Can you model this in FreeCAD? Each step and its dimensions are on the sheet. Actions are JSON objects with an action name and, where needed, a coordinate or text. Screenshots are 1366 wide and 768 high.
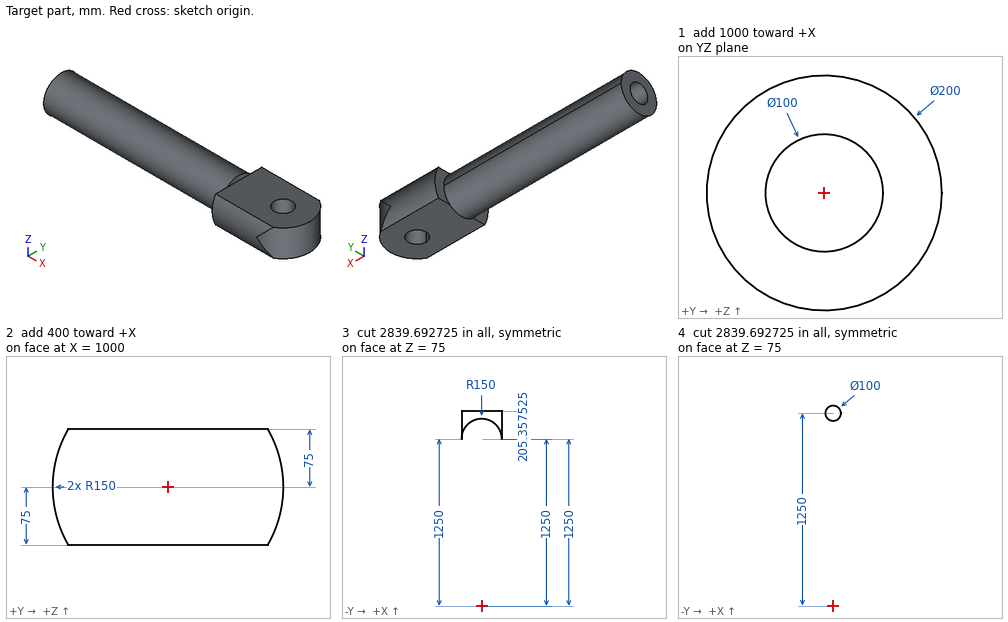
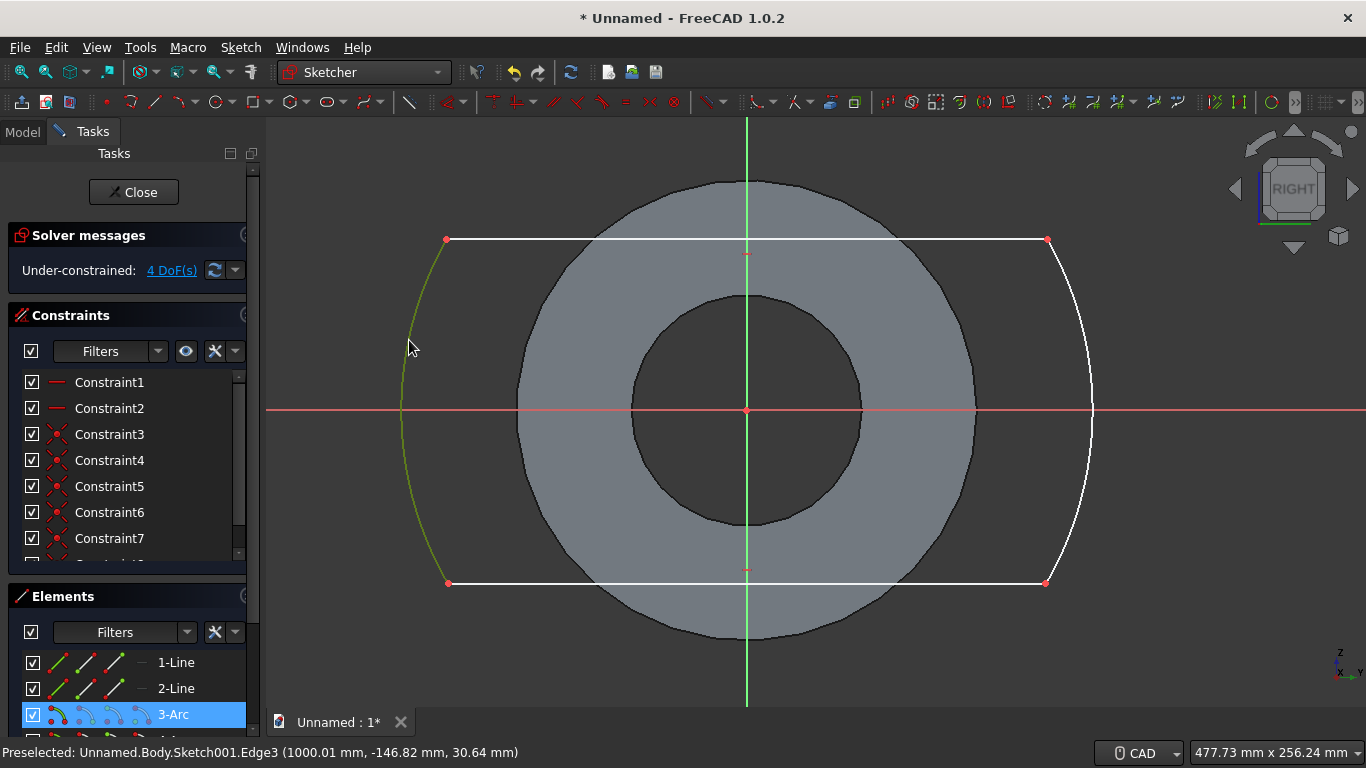
{"action": "left_click", "coordinate": [1085, 483]}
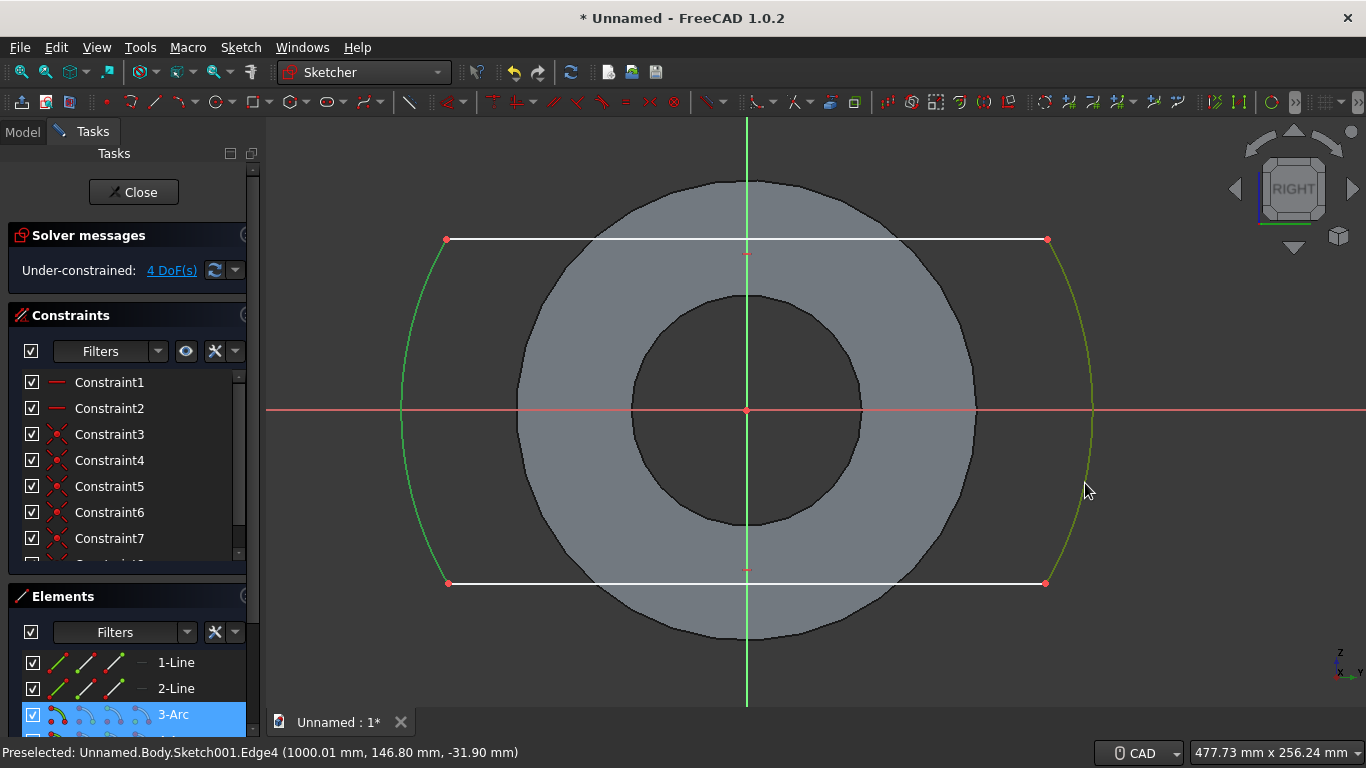
{"action": "left_click", "coordinate": [626, 102]}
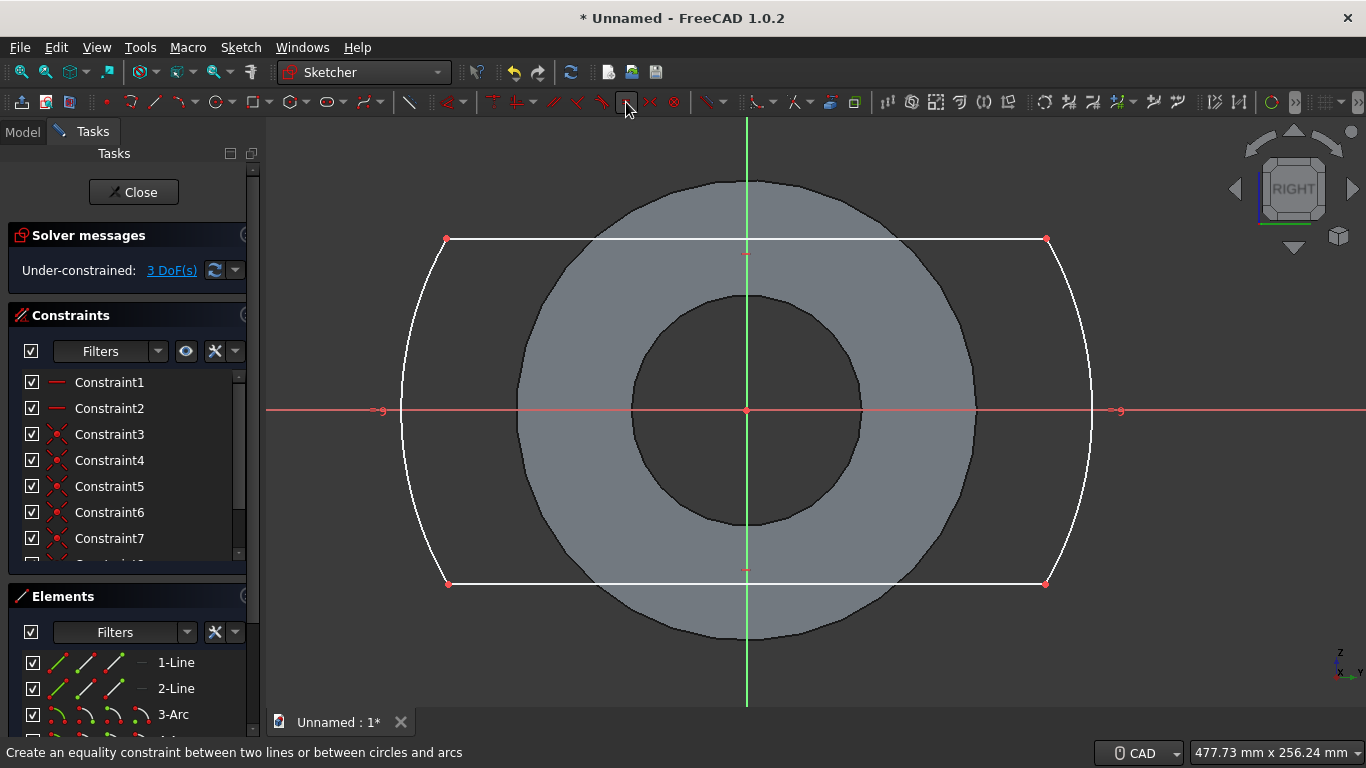
{"action": "left_click", "coordinate": [448, 102]}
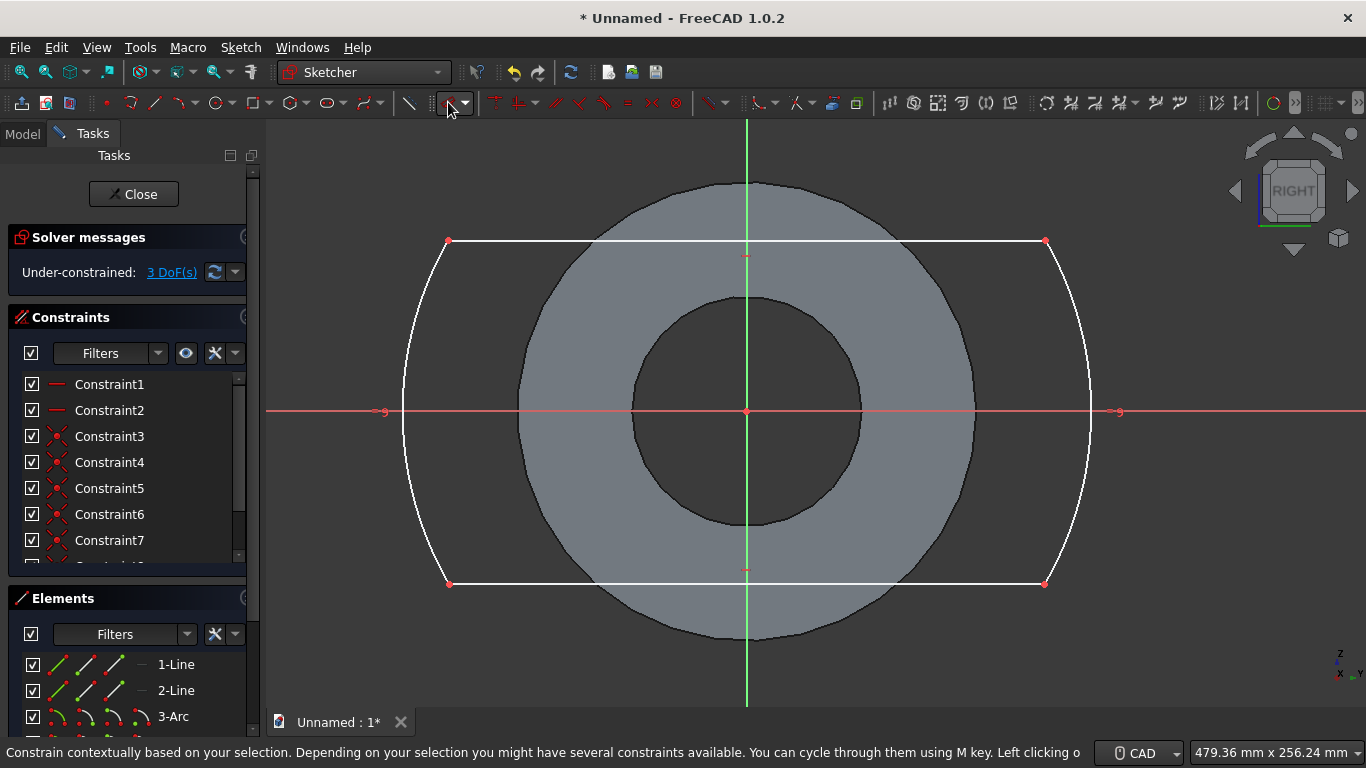
{"action": "left_click", "coordinate": [410, 341]}
{"action": "left_click", "coordinate": [379, 334]}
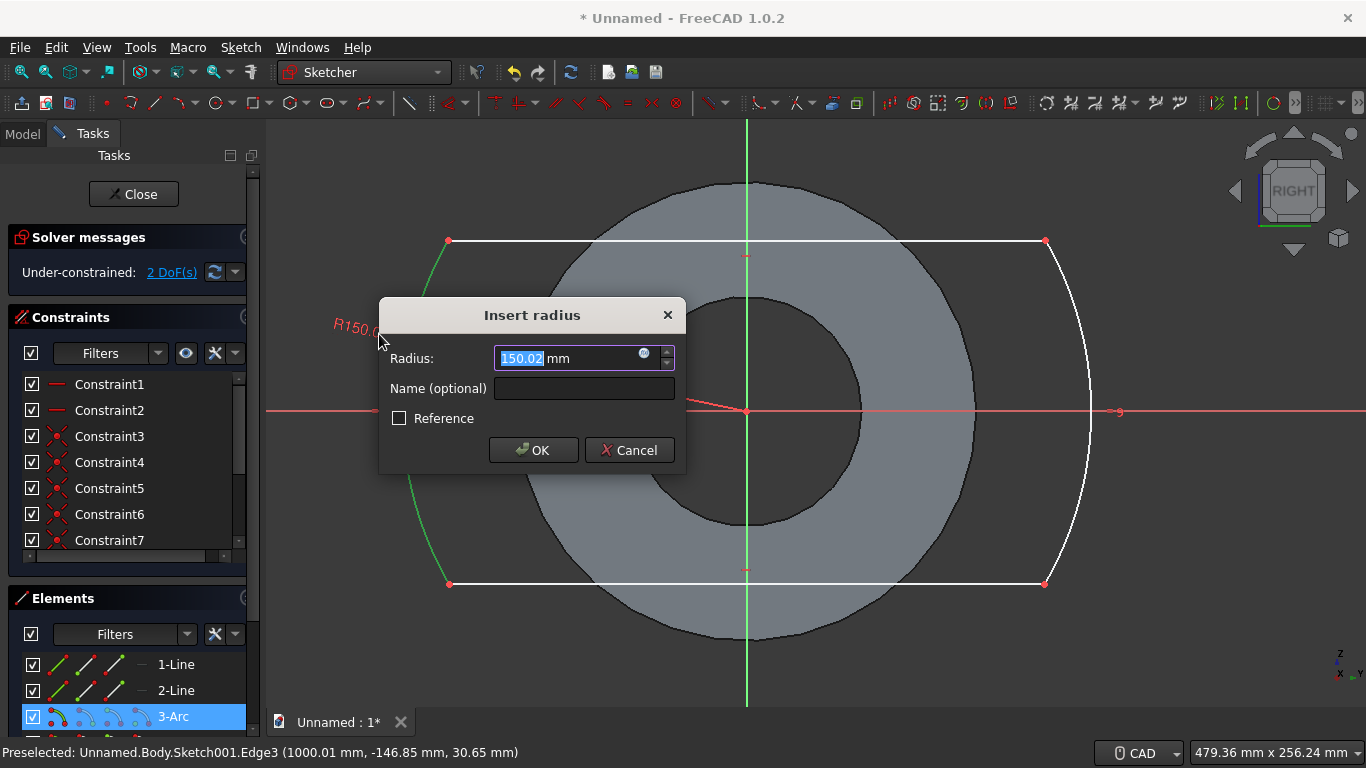
{"action": "type", "text": "150"}
{"action": "key", "text": "Return"}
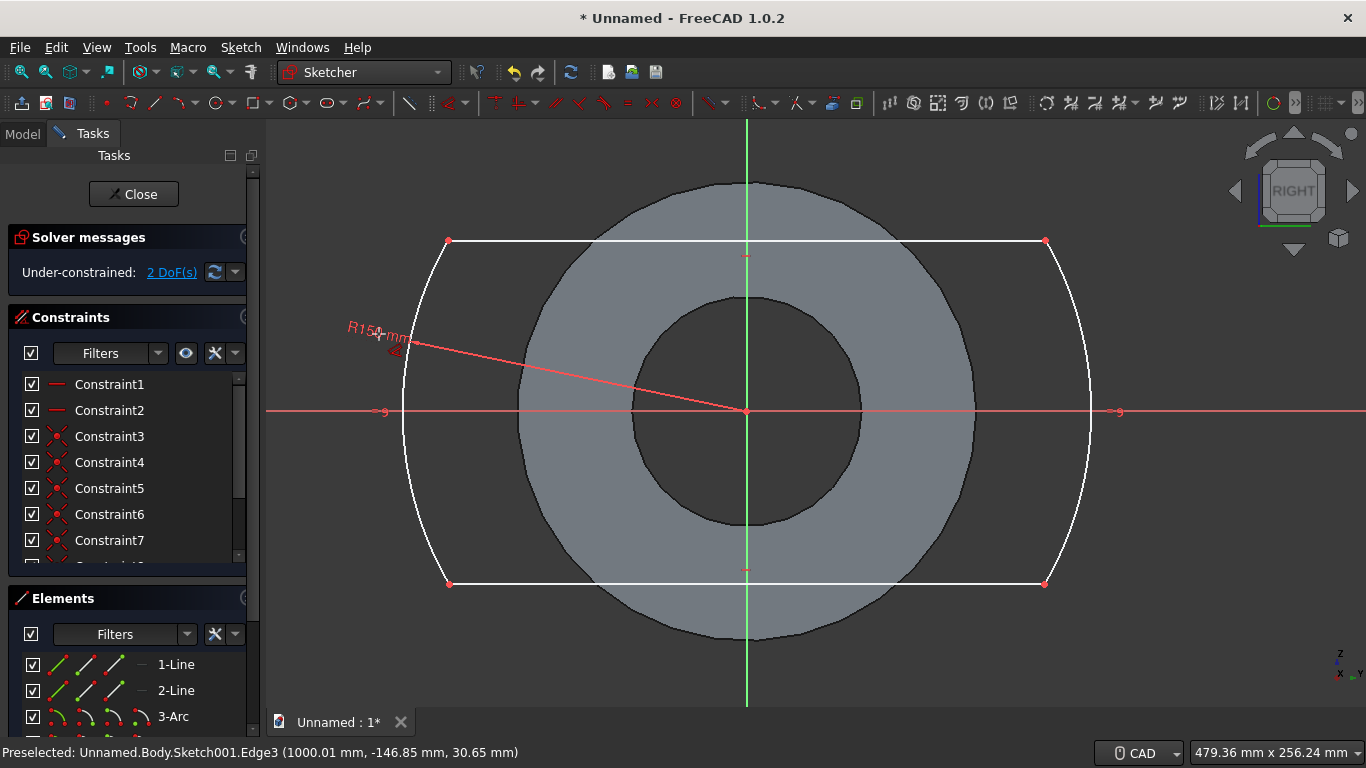
{"action": "left_click", "coordinate": [1046, 241]}
{"action": "left_click", "coordinate": [1080, 266]}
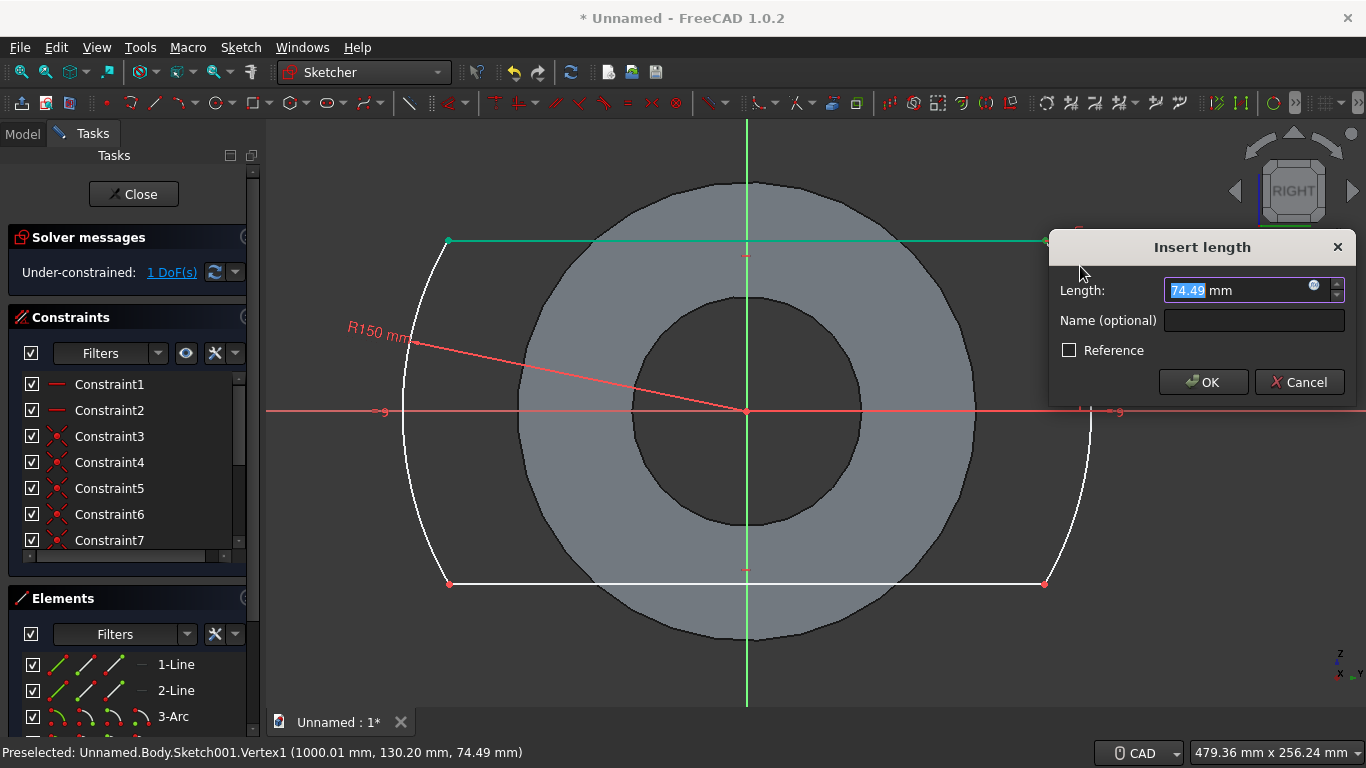
{"action": "type", "text": "75"}
{"action": "key", "text": "Return"}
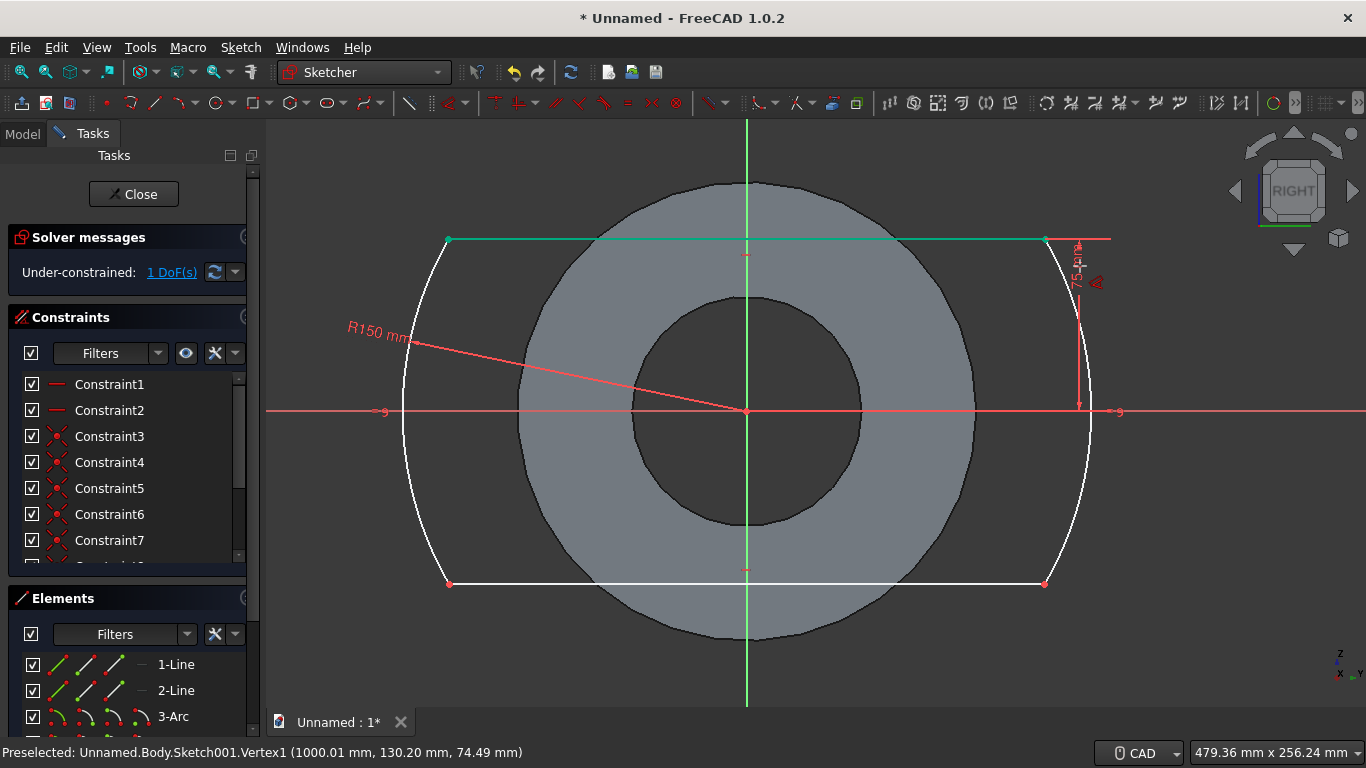
{"action": "left_click", "coordinate": [449, 584]}
{"action": "left_click", "coordinate": [415, 559]}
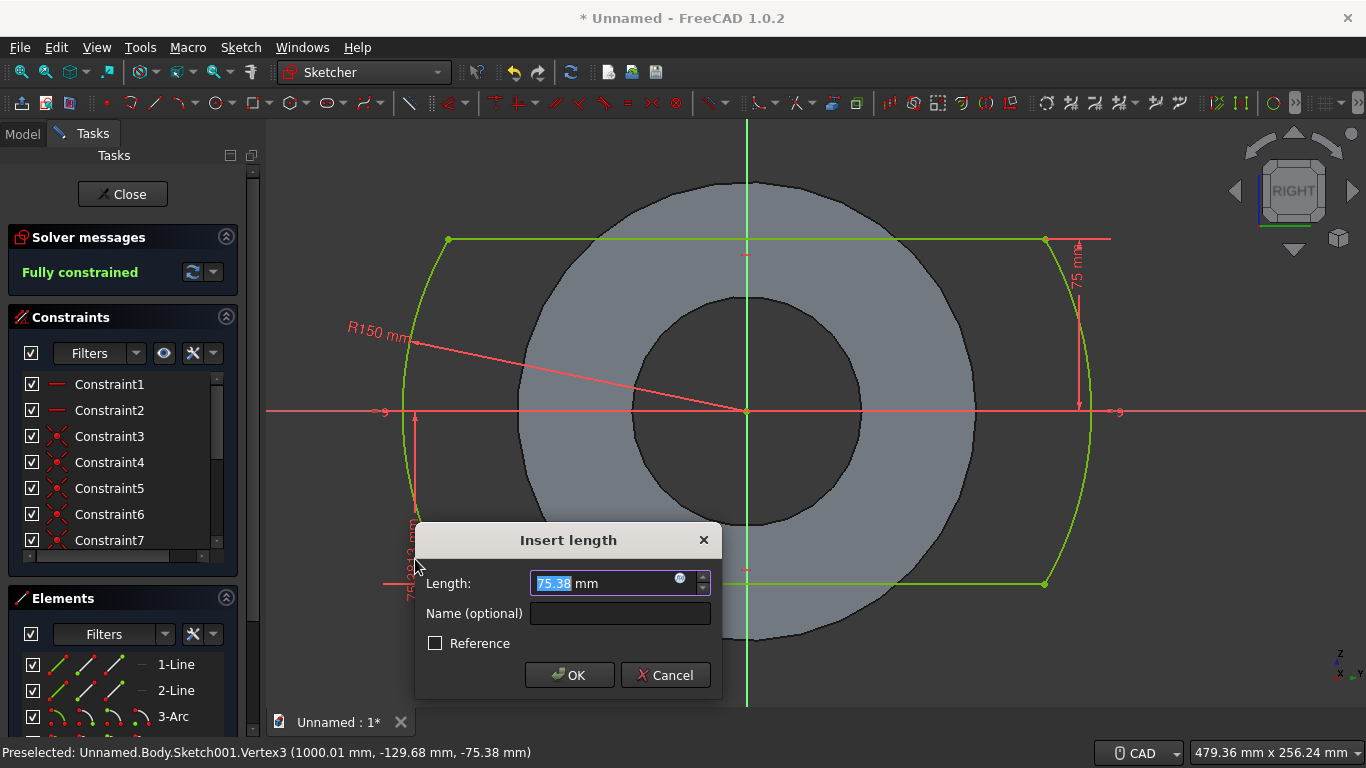
{"action": "type", "text": "75"}
{"action": "key", "text": "Return"}
{"action": "key", "text": "Escape"}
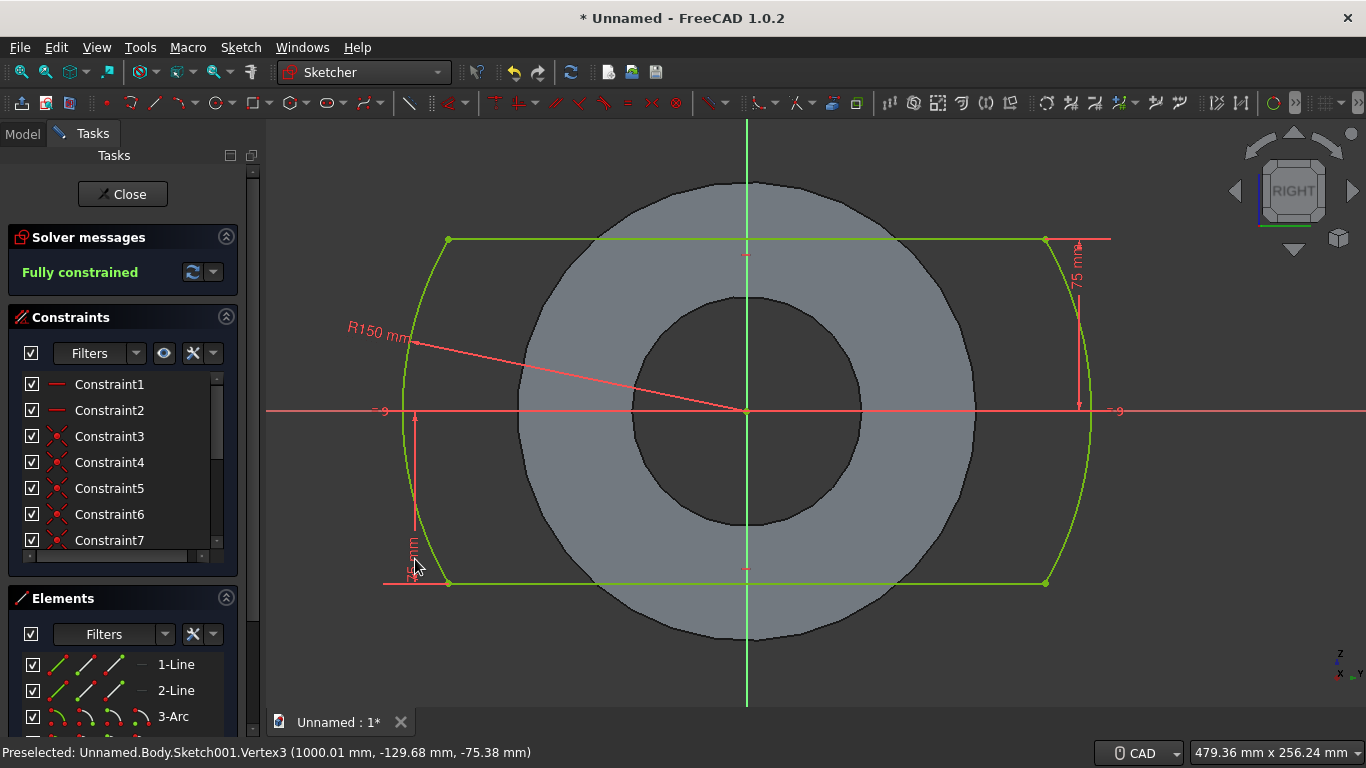
{"action": "left_click", "coordinate": [123, 194]}